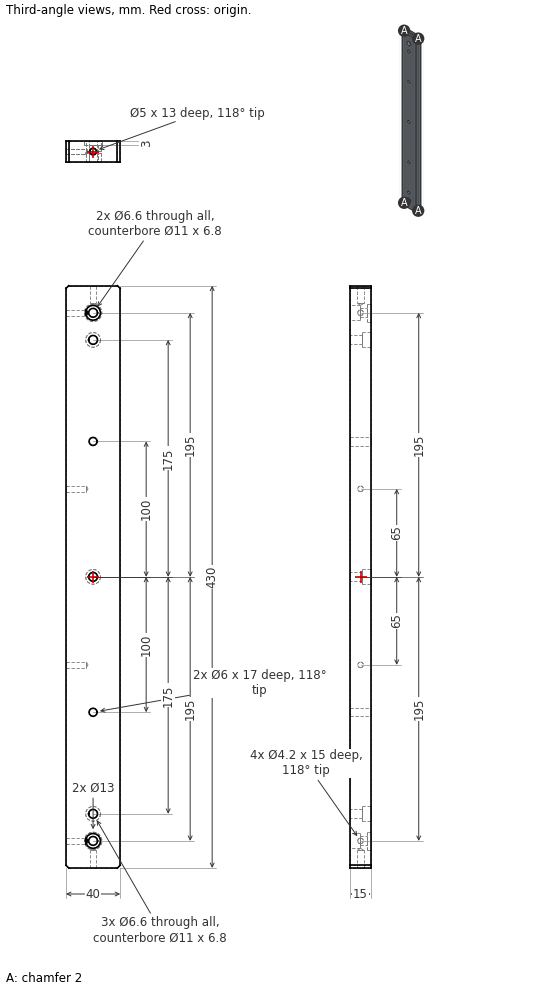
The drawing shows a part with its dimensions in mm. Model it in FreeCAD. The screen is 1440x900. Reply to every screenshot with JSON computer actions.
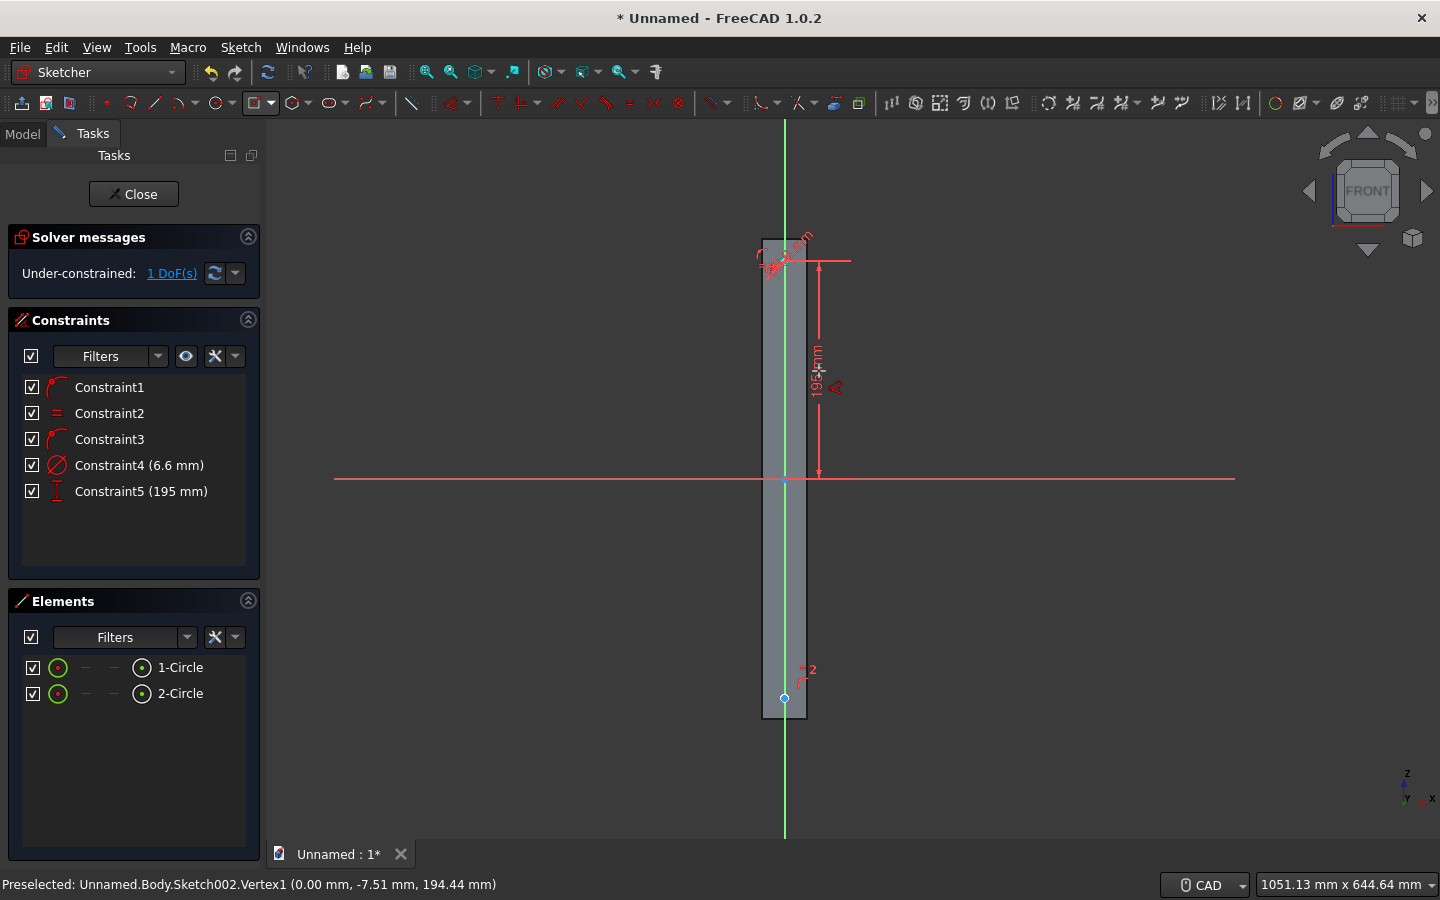
{"action": "left_click", "coordinate": [785, 698]}
{"action": "left_click", "coordinate": [819, 589]}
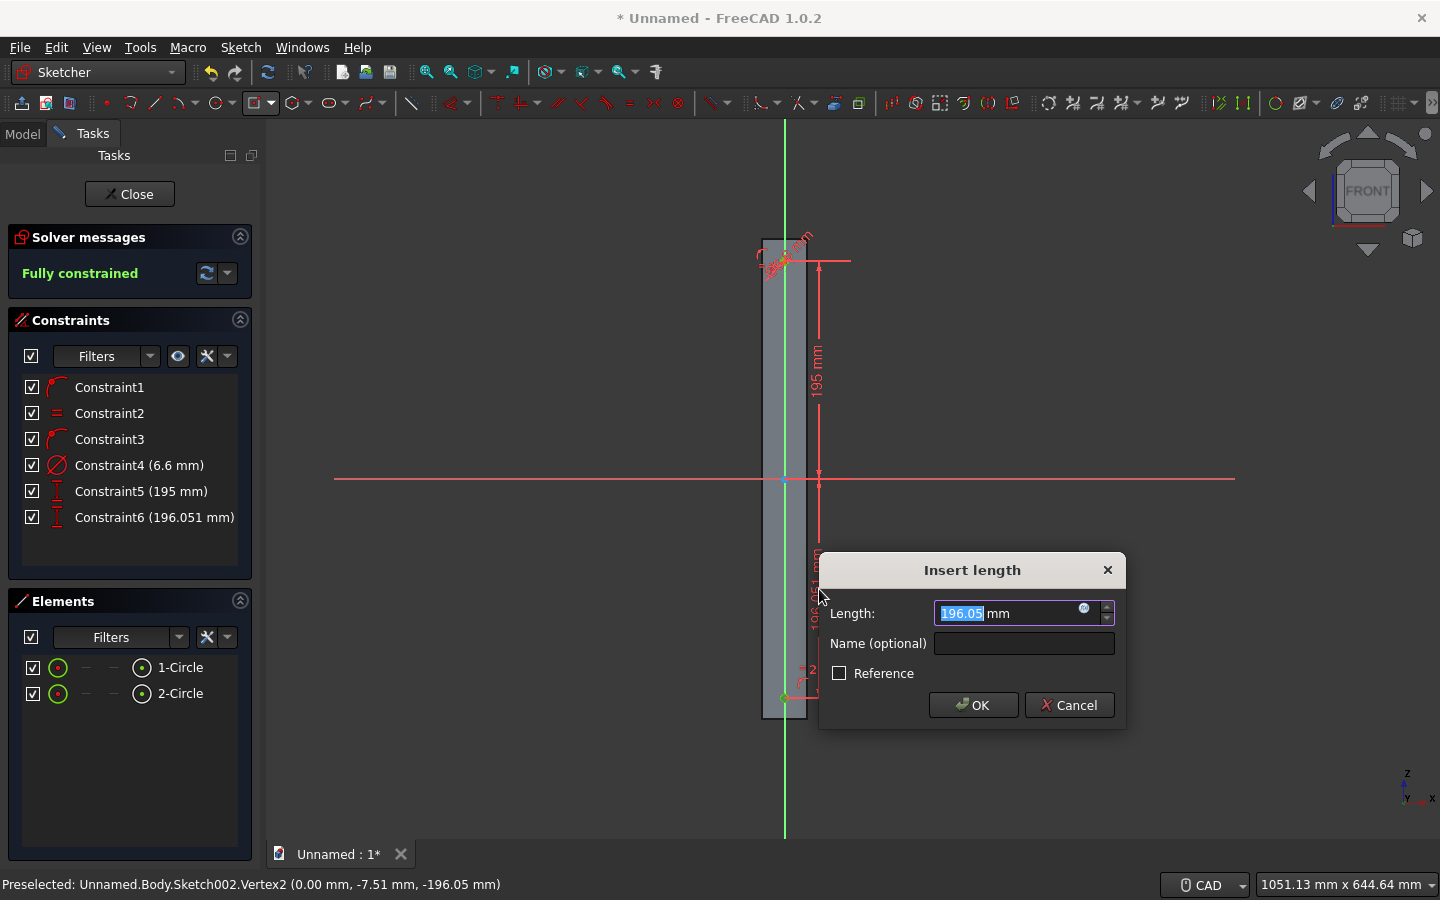
{"action": "type", "text": "195"}
{"action": "key", "text": "Return"}
{"action": "key", "text": "Escape"}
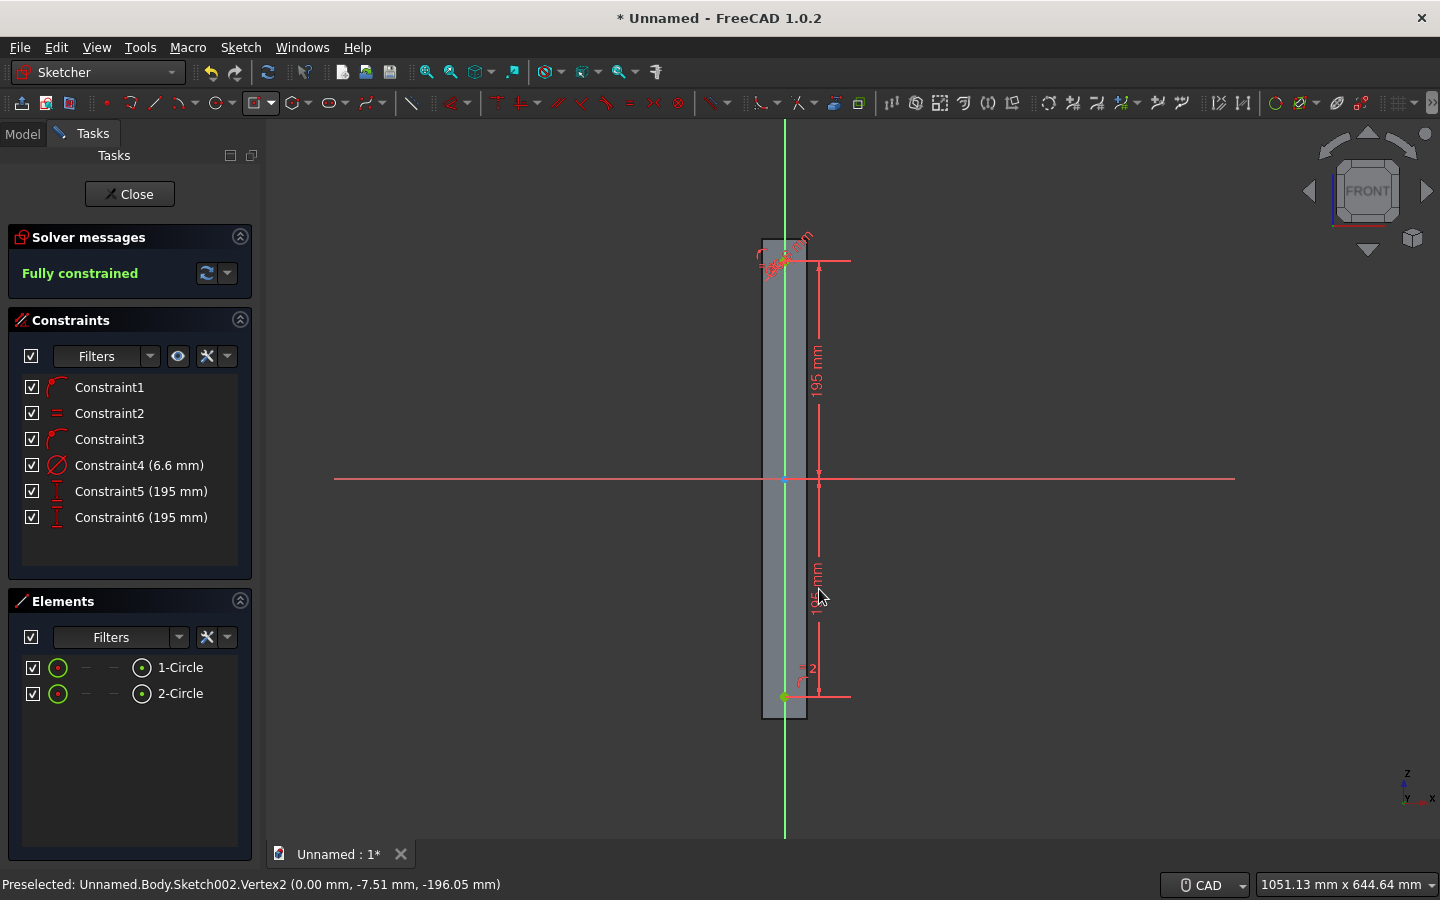
{"action": "left_click", "coordinate": [130, 194]}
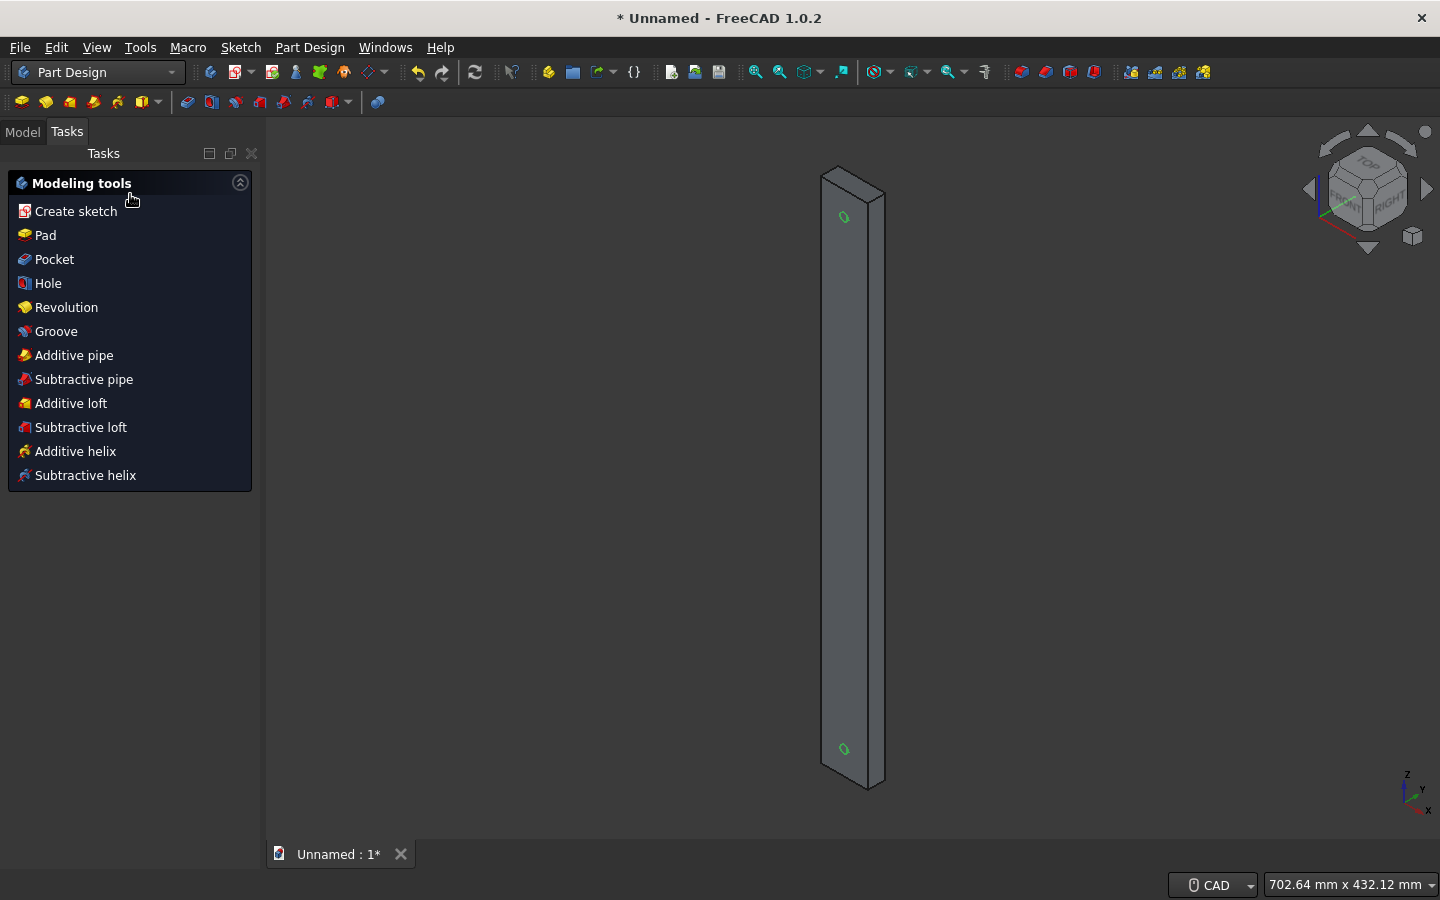
{"action": "left_click", "coordinate": [212, 102]}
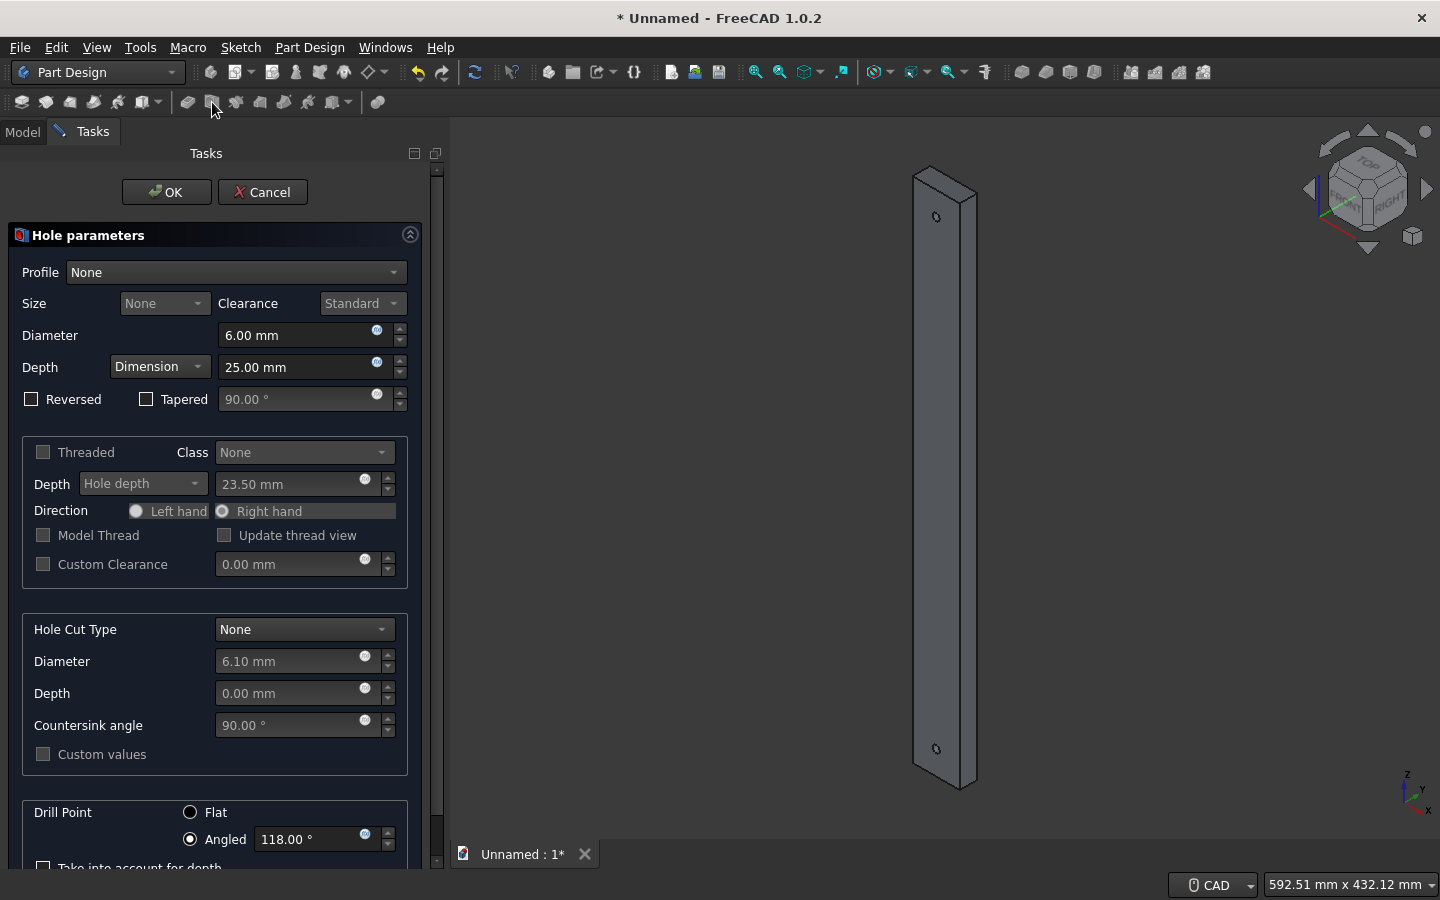
{"action": "triple_click", "coordinate": [305, 335]}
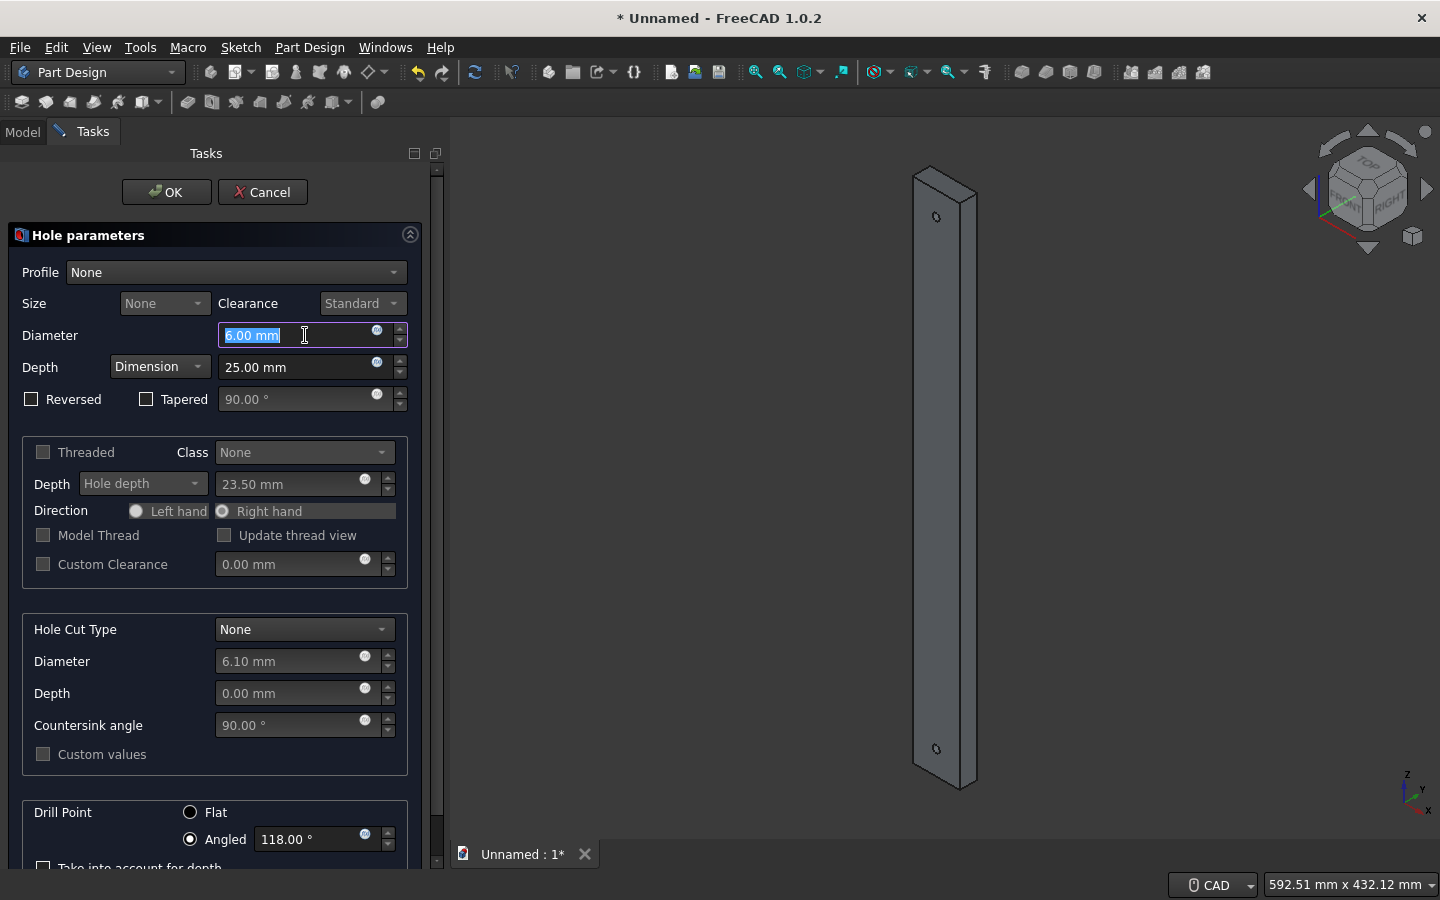
{"action": "type", "text": "6.6"}
{"action": "key", "text": "Tab"}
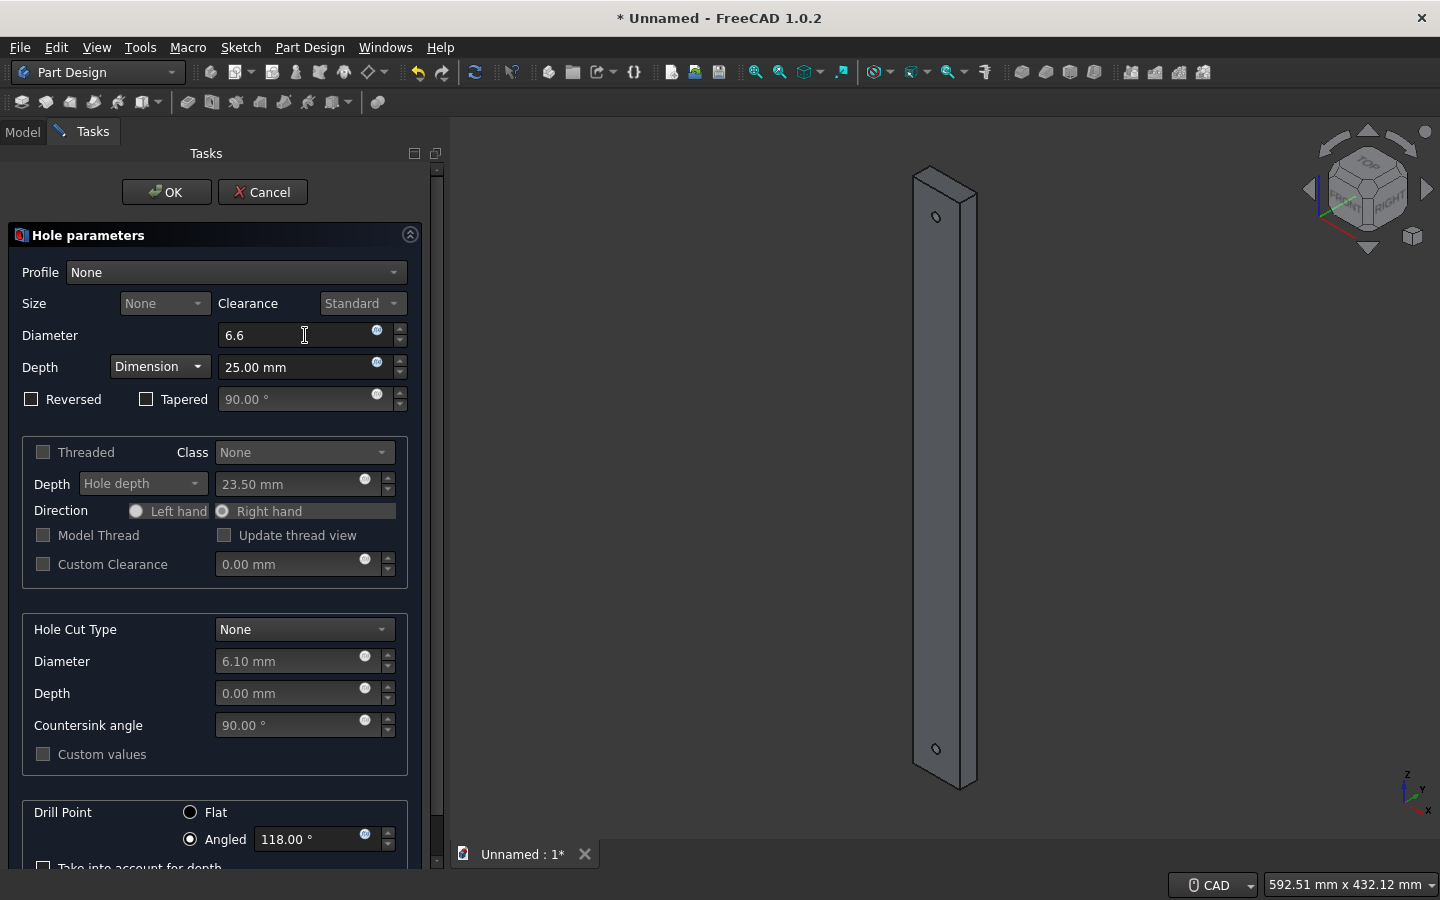
{"action": "left_click", "coordinate": [161, 366]}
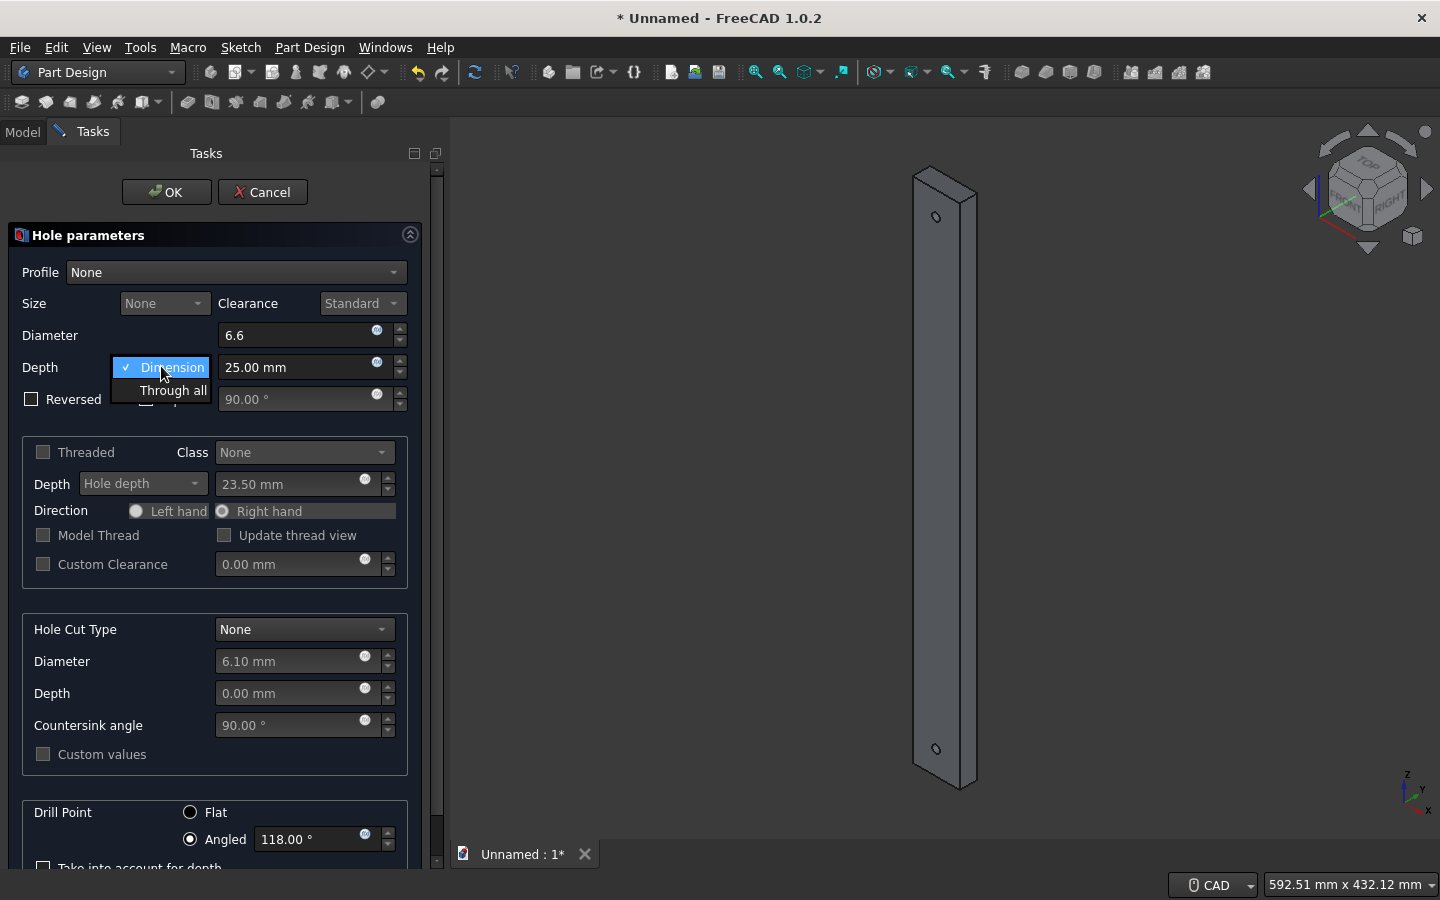
{"action": "left_click", "coordinate": [160, 390]}